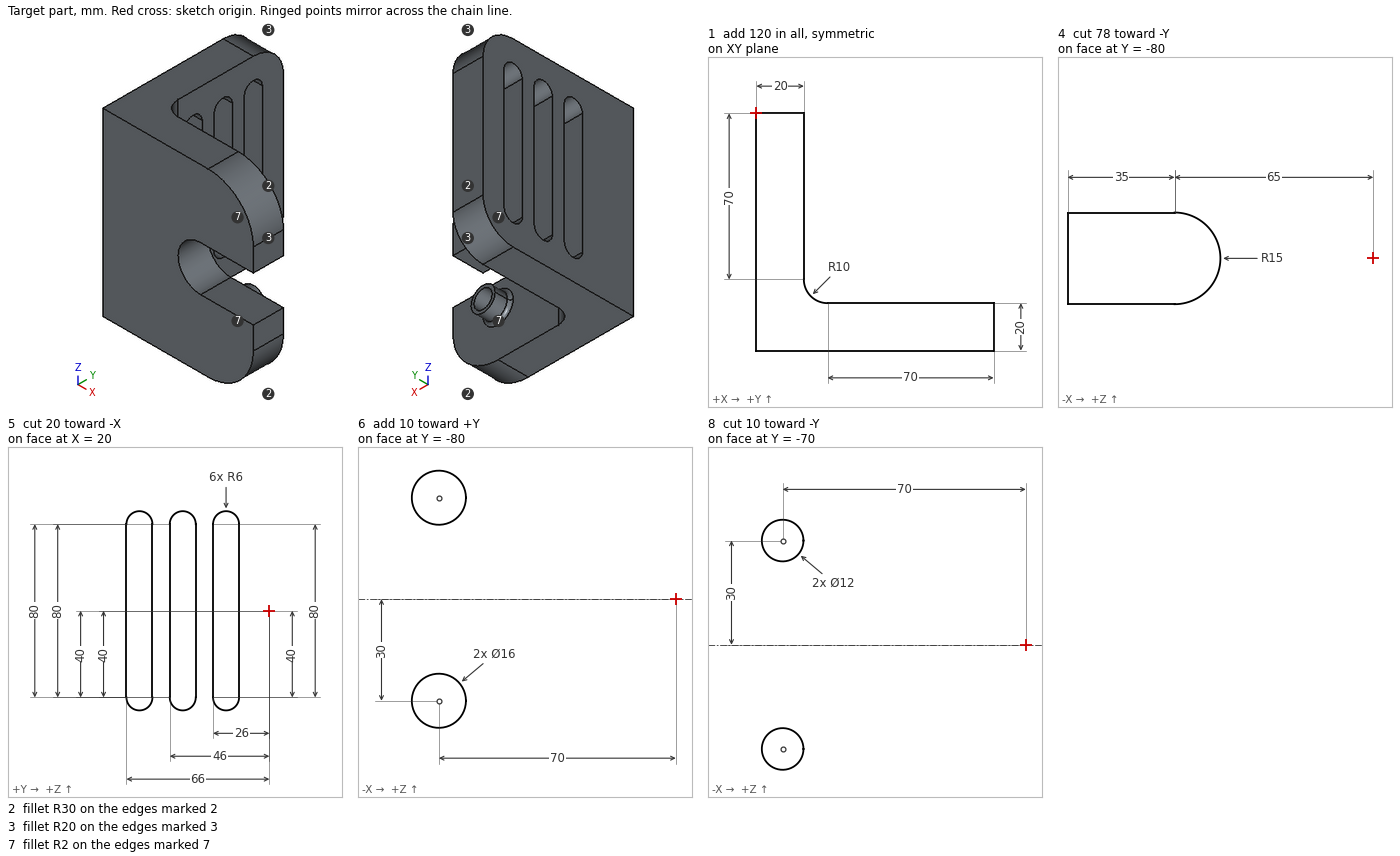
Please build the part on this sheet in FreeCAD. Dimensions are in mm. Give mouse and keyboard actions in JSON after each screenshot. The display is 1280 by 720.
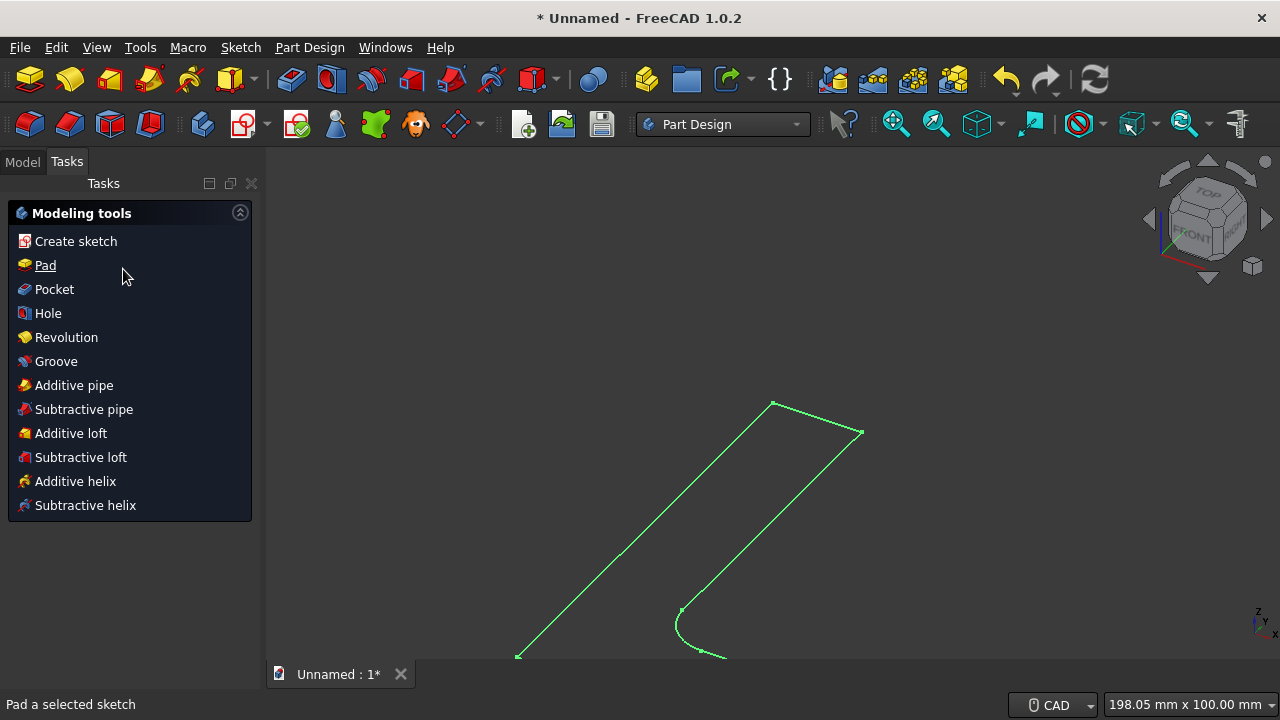
{"action": "left_click", "coordinate": [30, 80]}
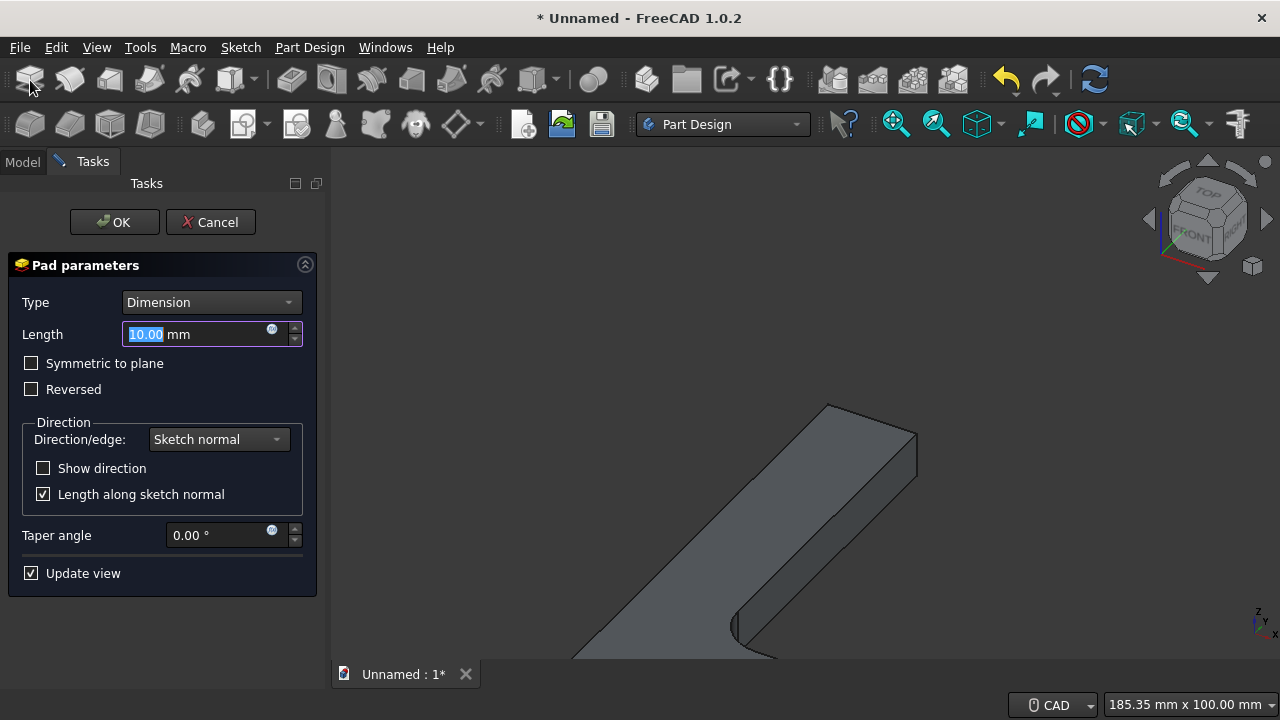
{"action": "type", "text": "120"}
{"action": "key", "text": "Tab"}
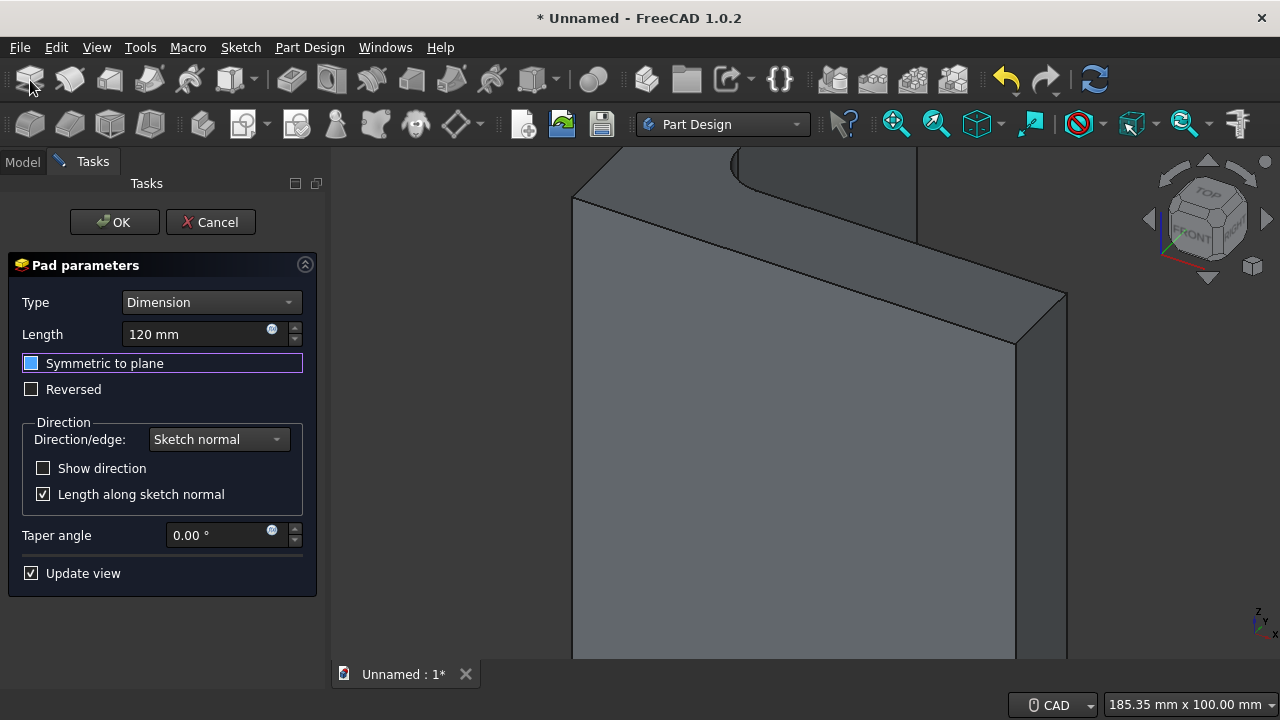
{"action": "left_click", "coordinate": [30, 363]}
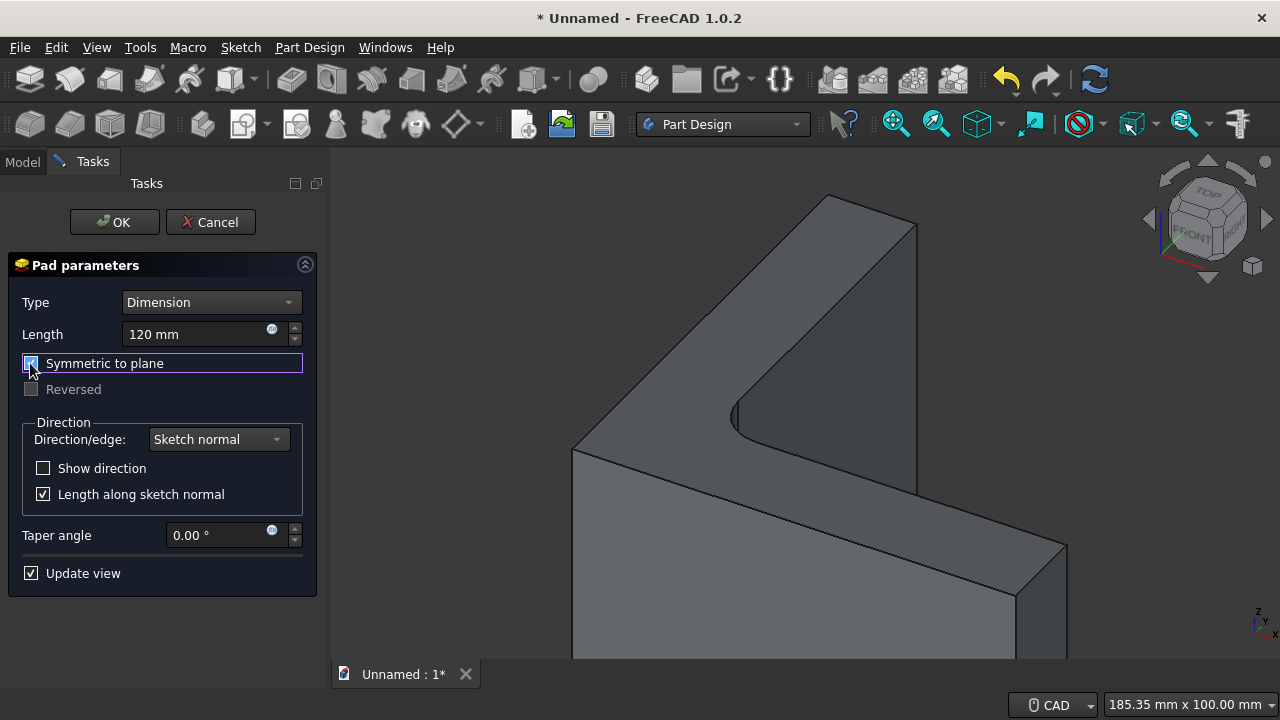
{"action": "left_click", "coordinate": [115, 222]}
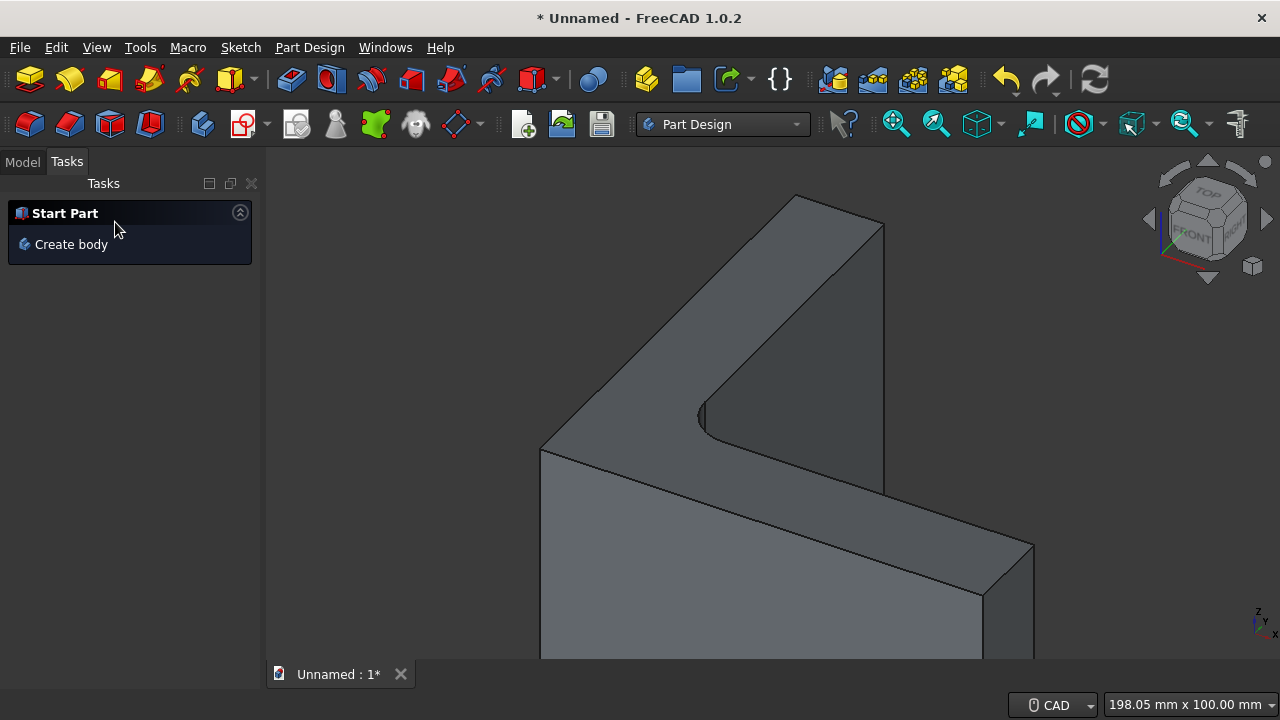
{"action": "left_click", "coordinate": [898, 124]}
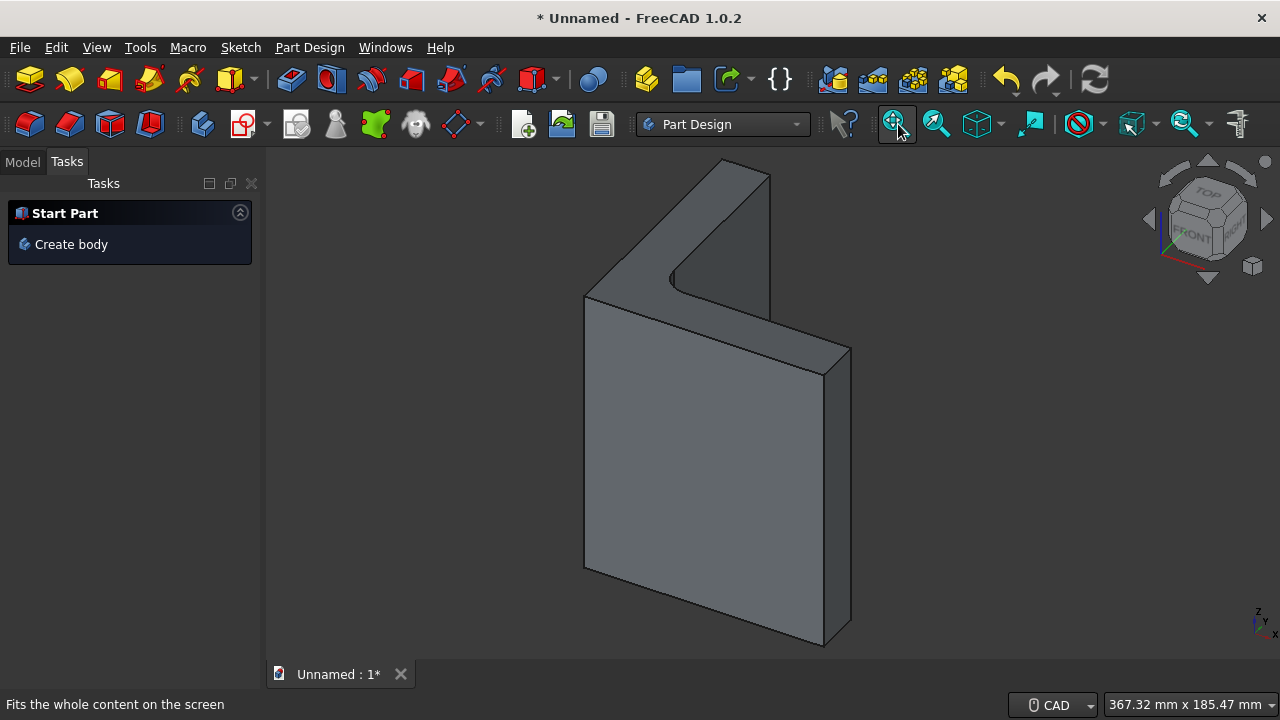
{"action": "left_click", "coordinate": [837, 361]}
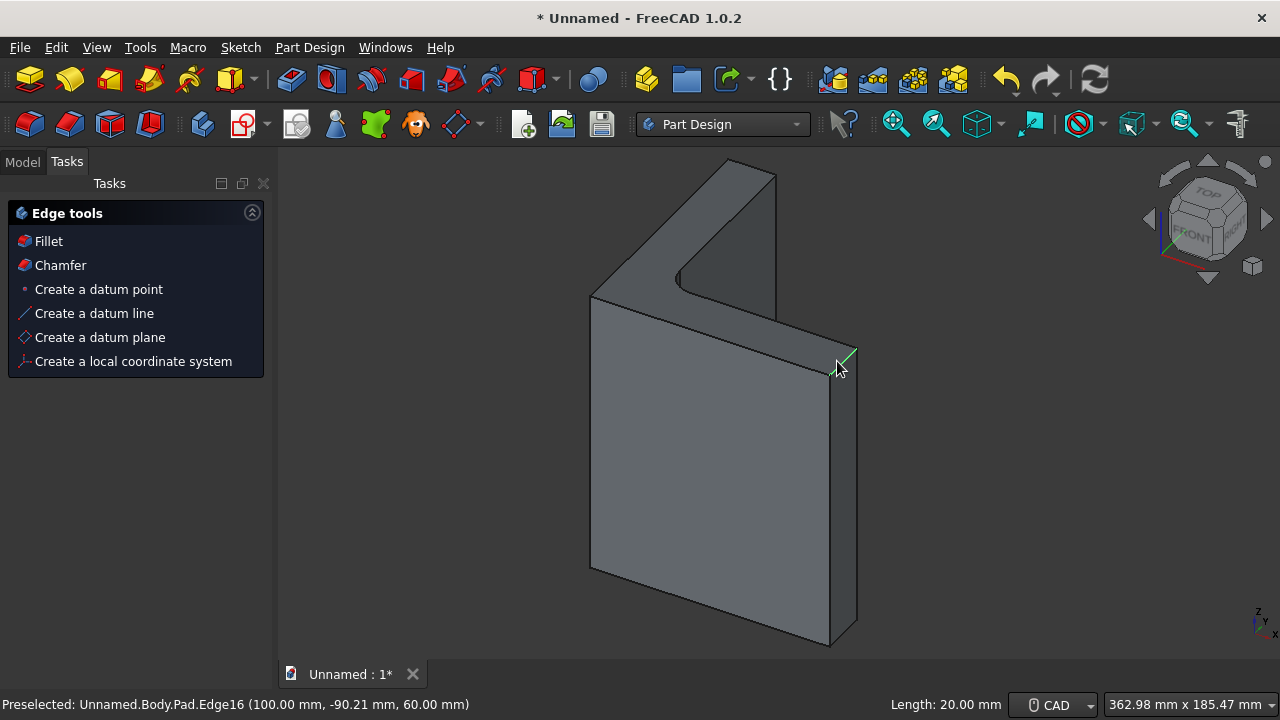
{"action": "key", "text": "0"}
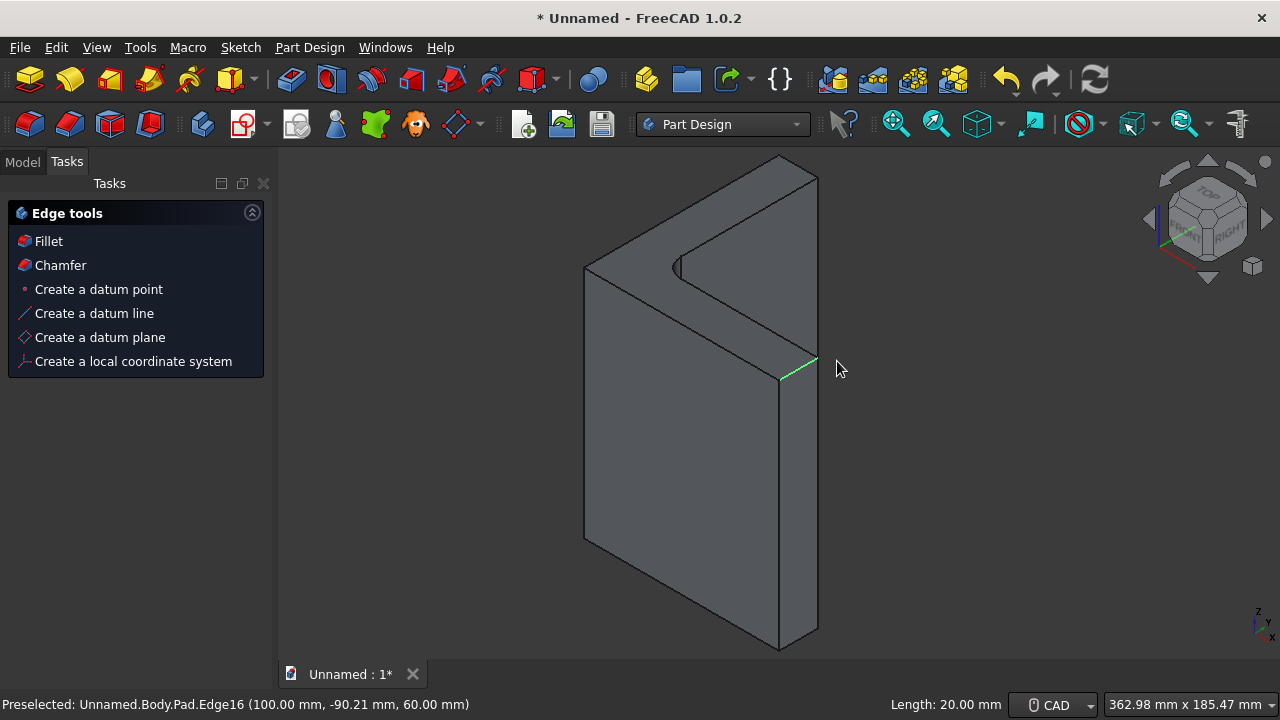
{"action": "key", "text": "2"}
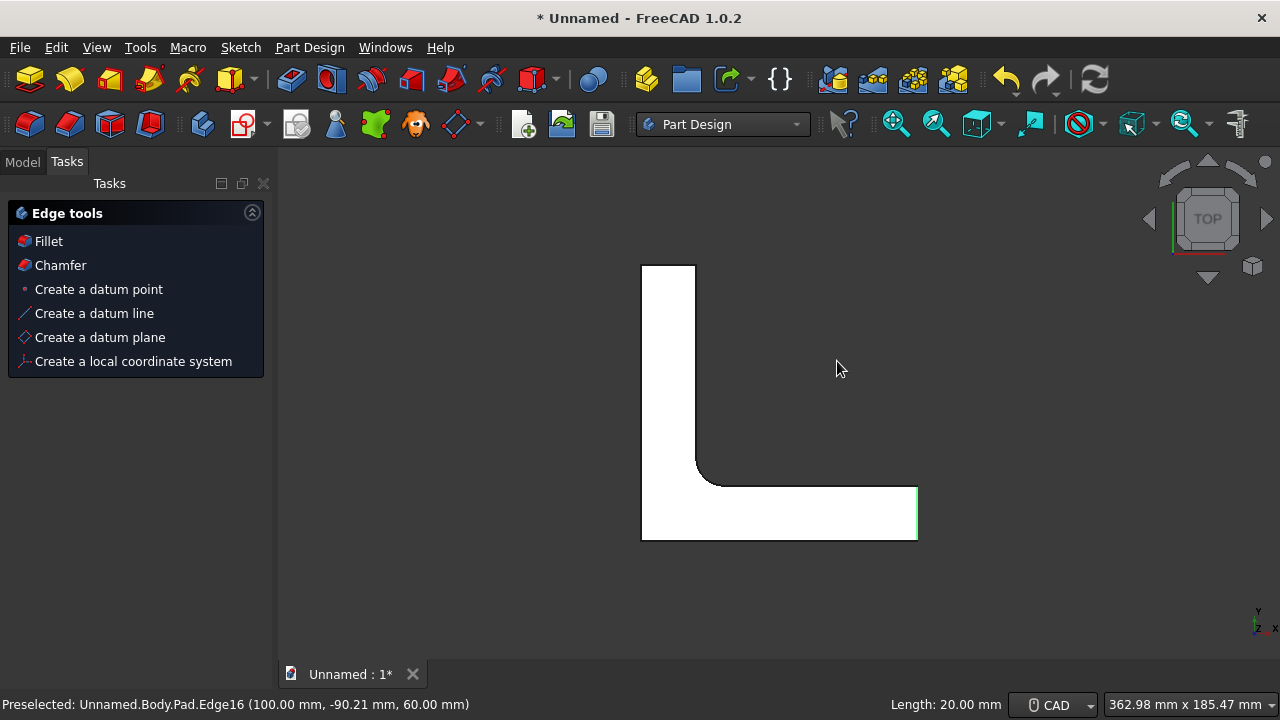
{"action": "key", "text": "1"}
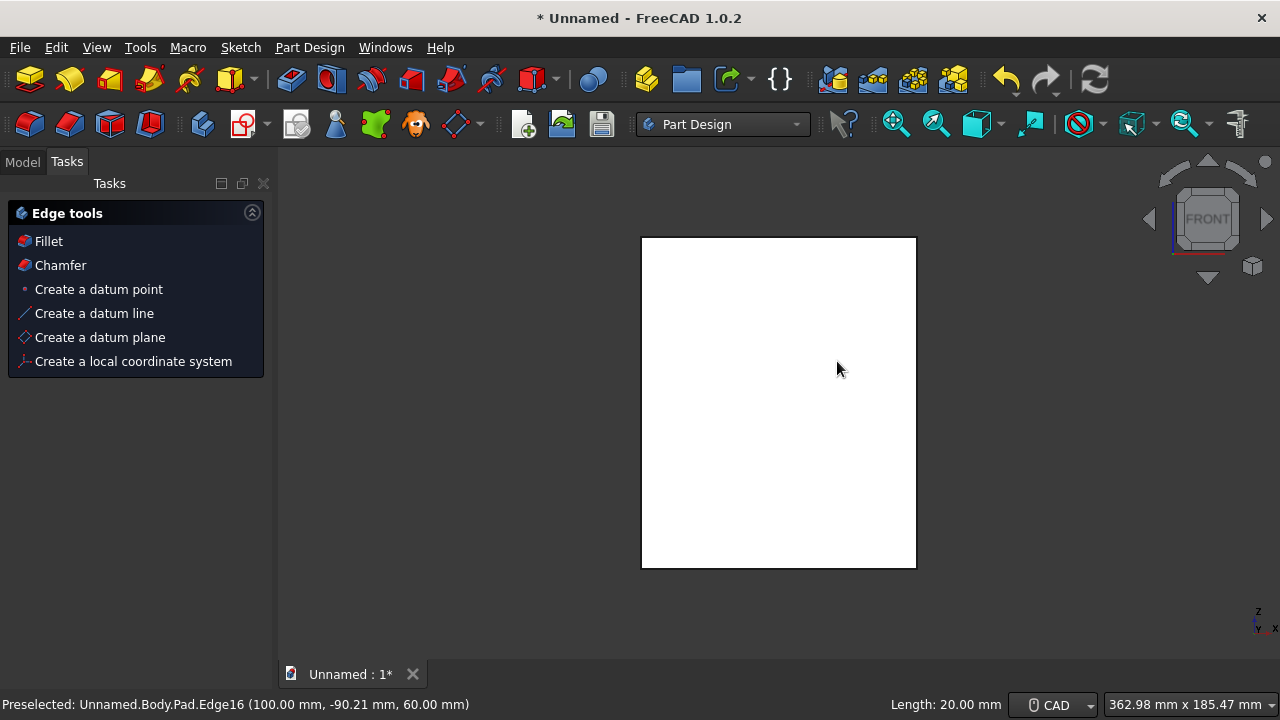
{"action": "key", "text": "3"}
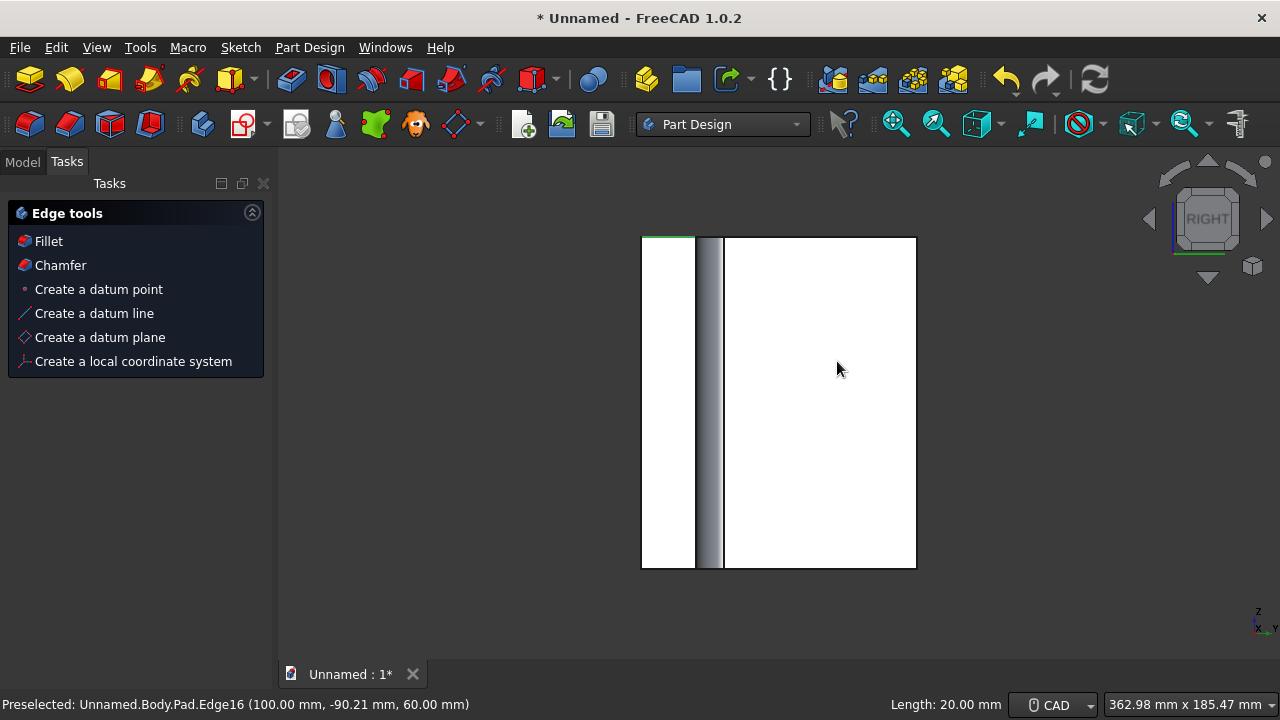
{"action": "left_click", "coordinate": [669, 568], "text": "ctrl"}